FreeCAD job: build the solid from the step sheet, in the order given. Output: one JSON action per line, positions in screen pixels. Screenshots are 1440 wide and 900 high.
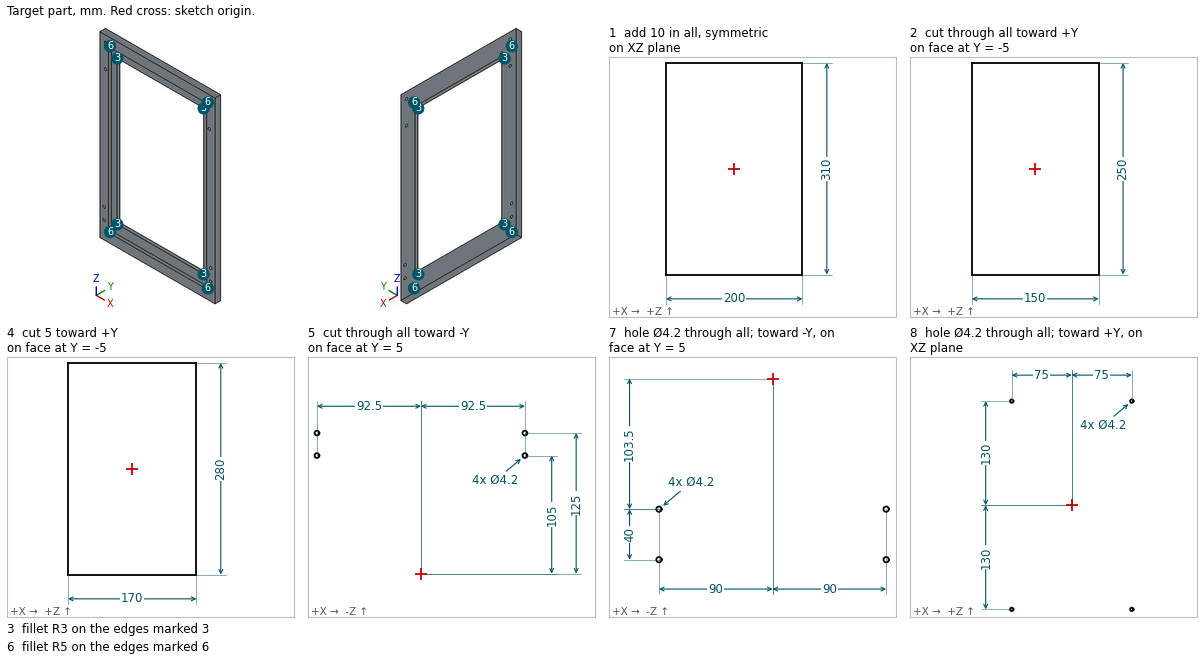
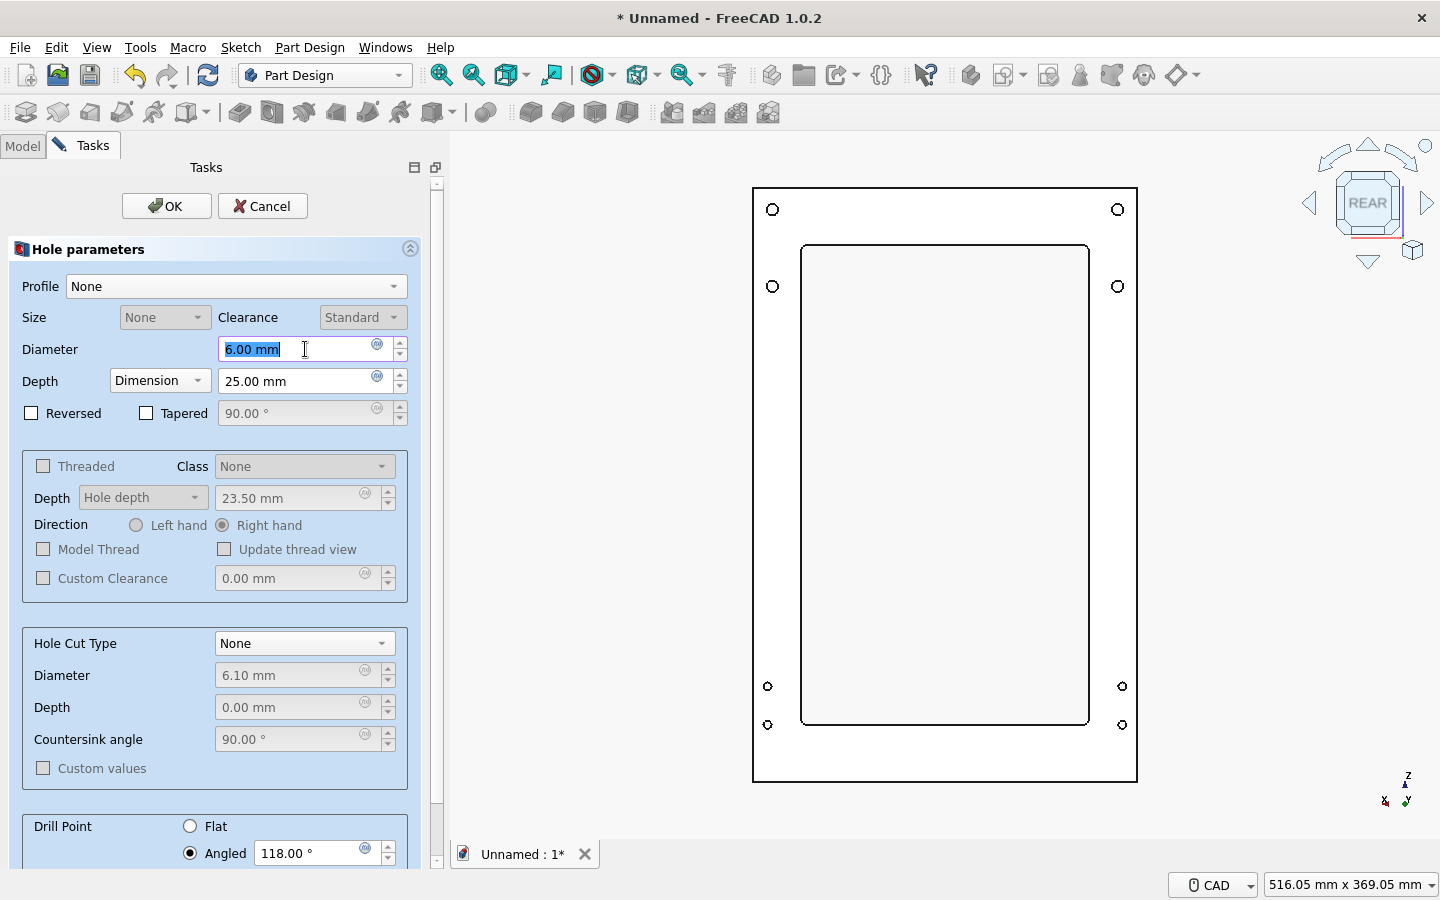
{"action": "type", "text": "4.2"}
{"action": "key", "text": "Tab"}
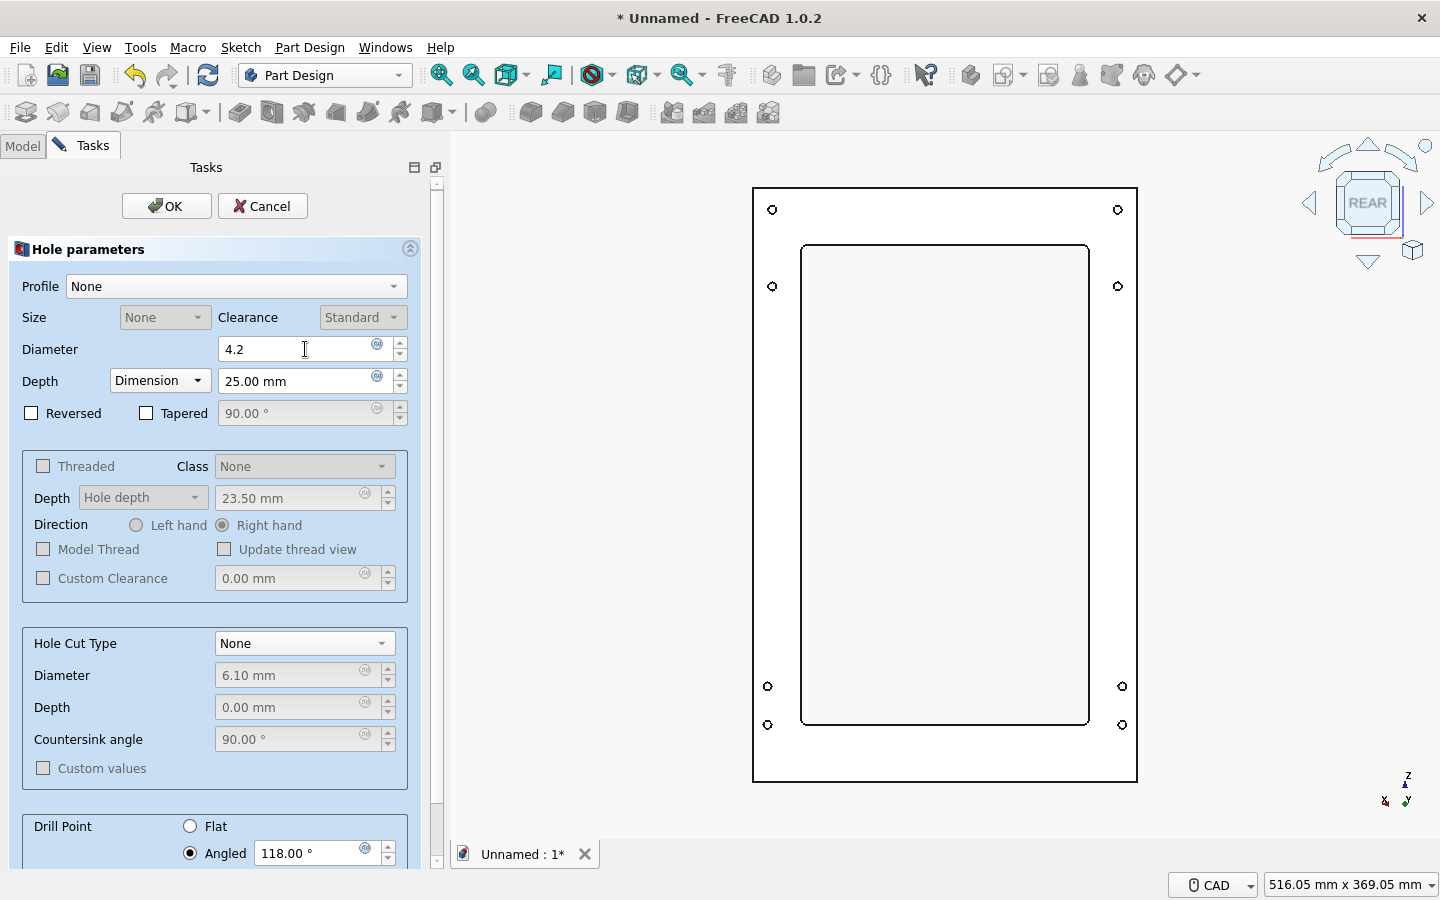
{"action": "left_click", "coordinate": [161, 380]}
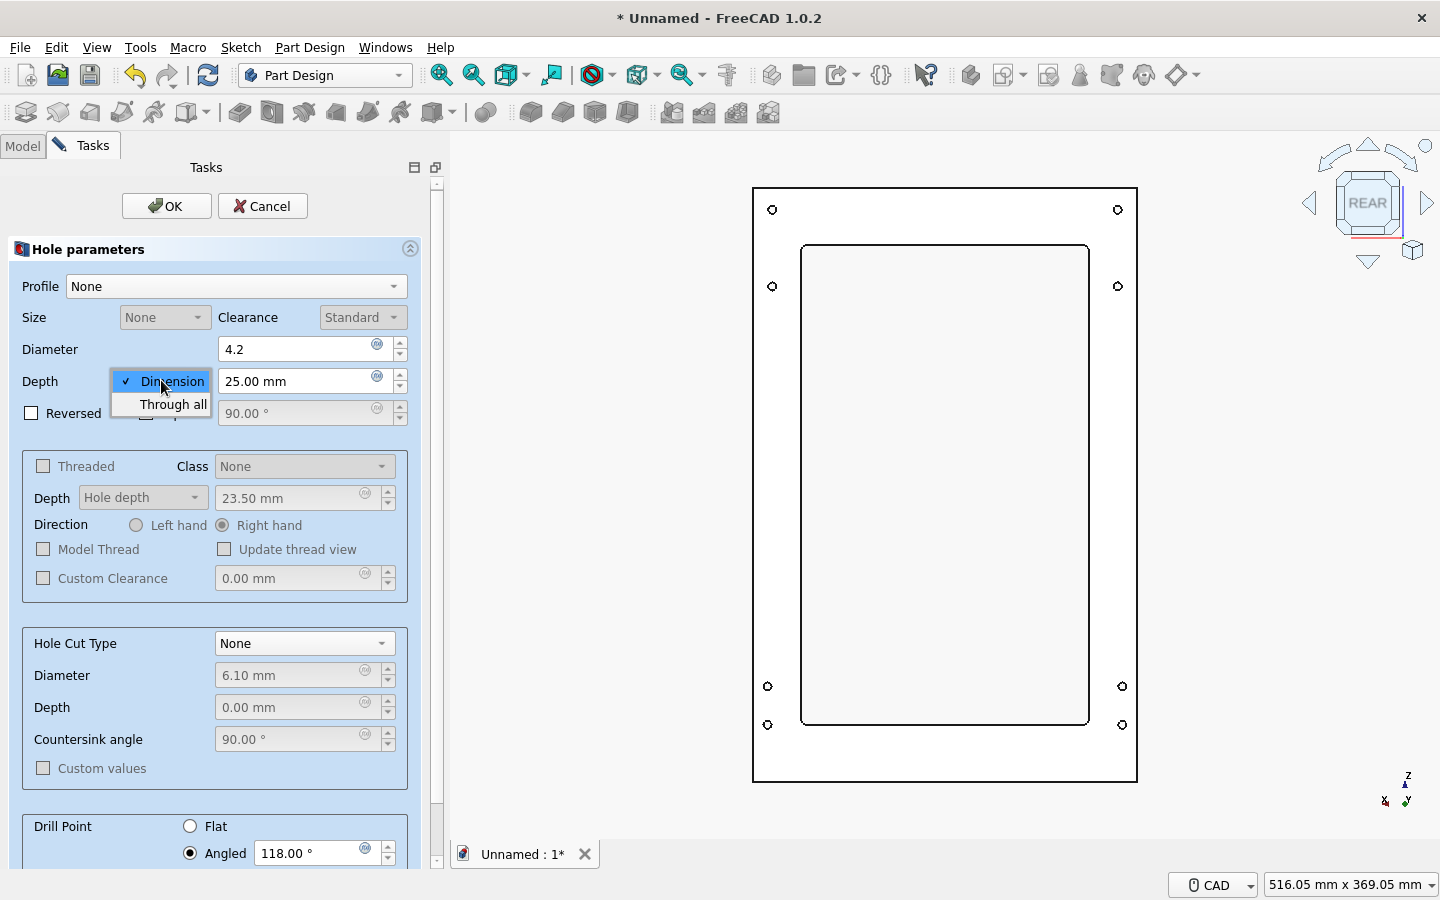
{"action": "left_click", "coordinate": [160, 404]}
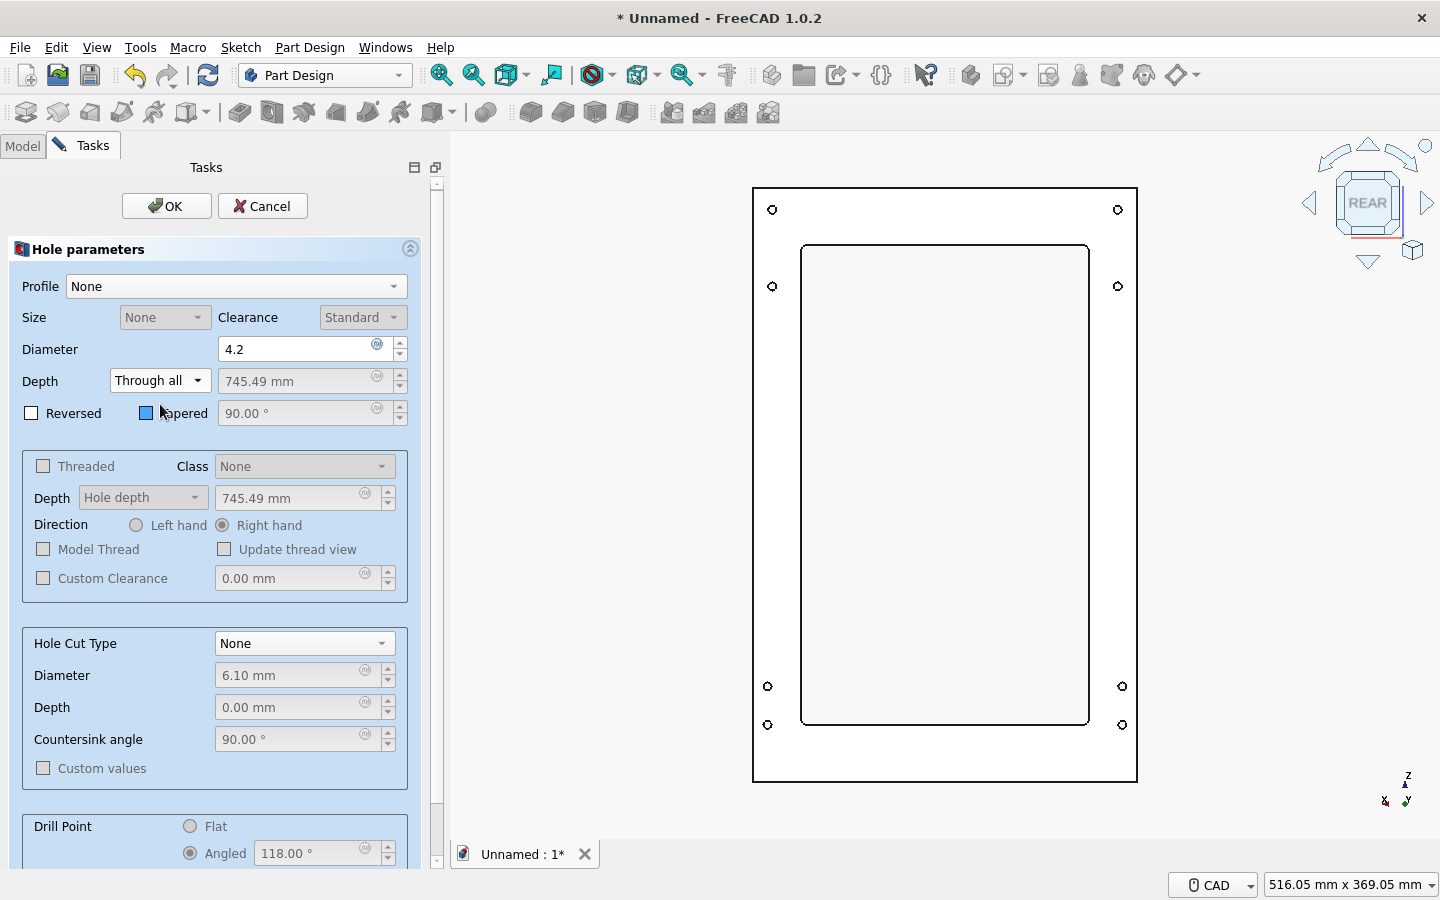
{"action": "left_click", "coordinate": [167, 206]}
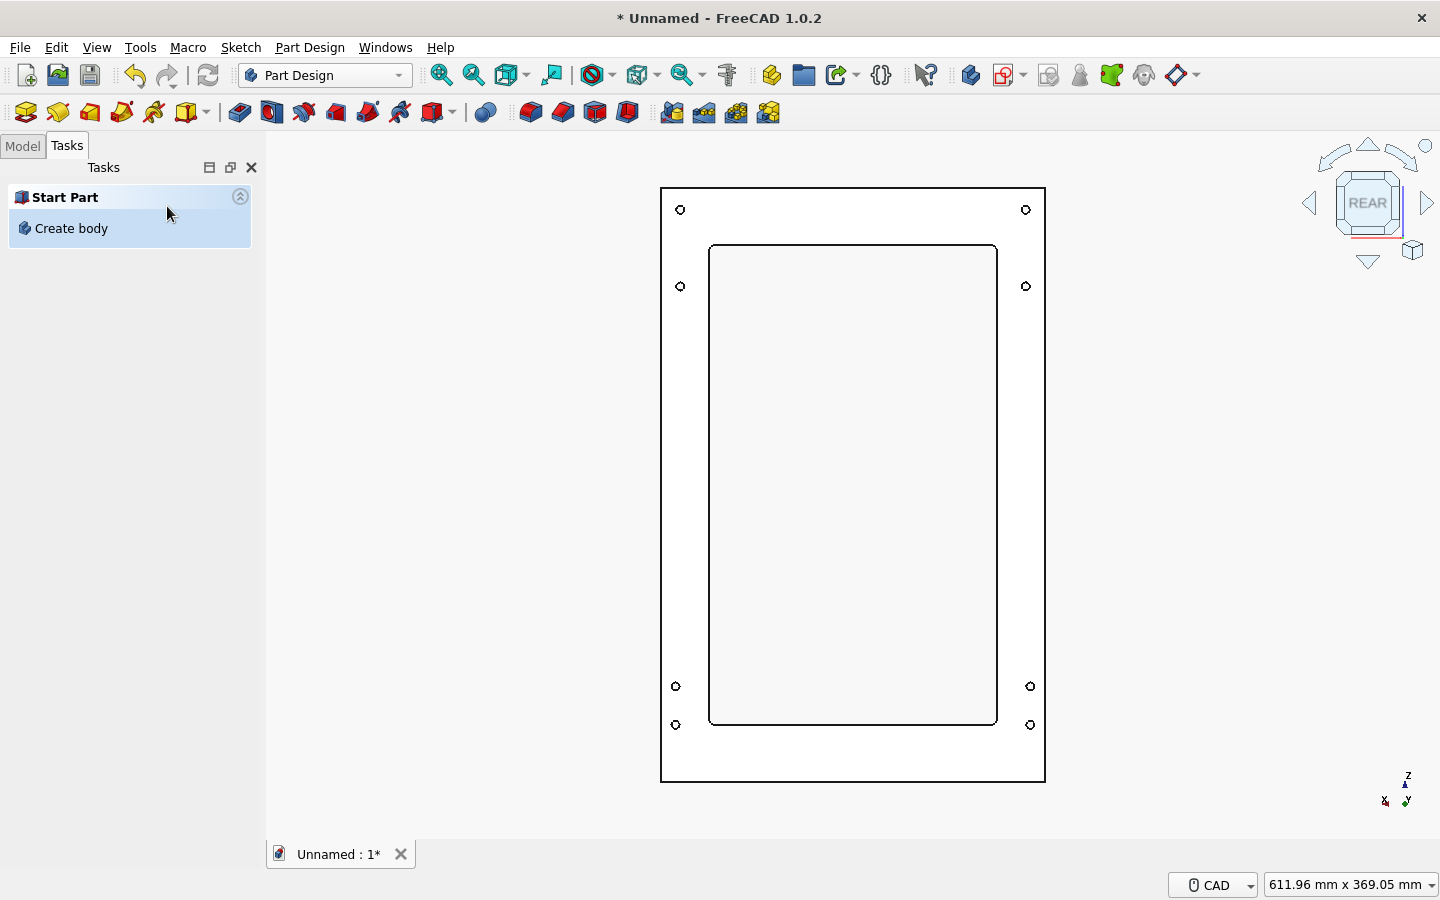
{"action": "left_click", "coordinate": [1004, 76]}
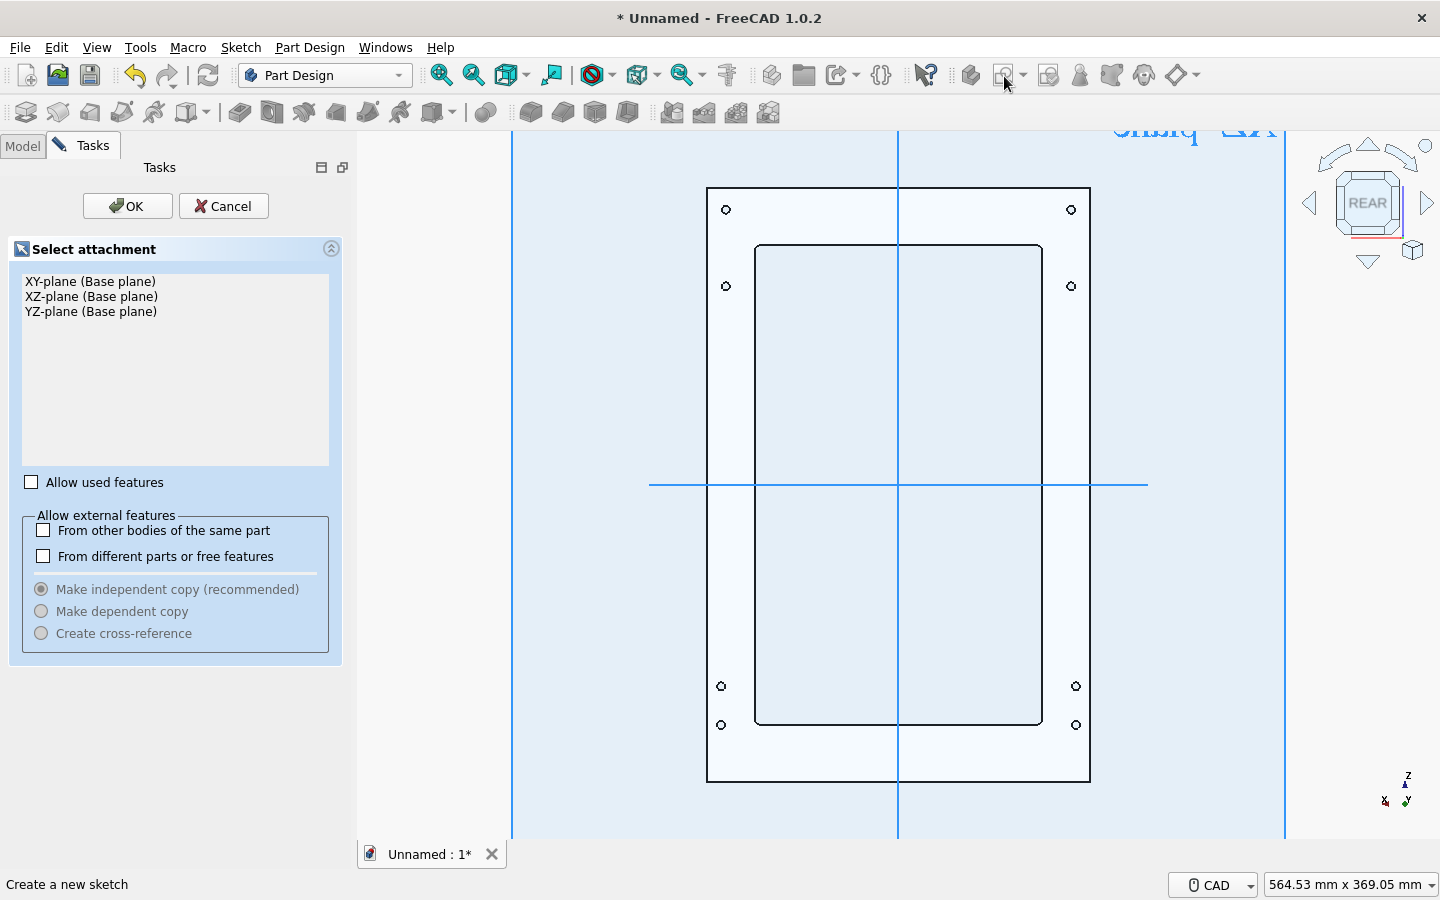
{"action": "left_click", "coordinate": [82, 296]}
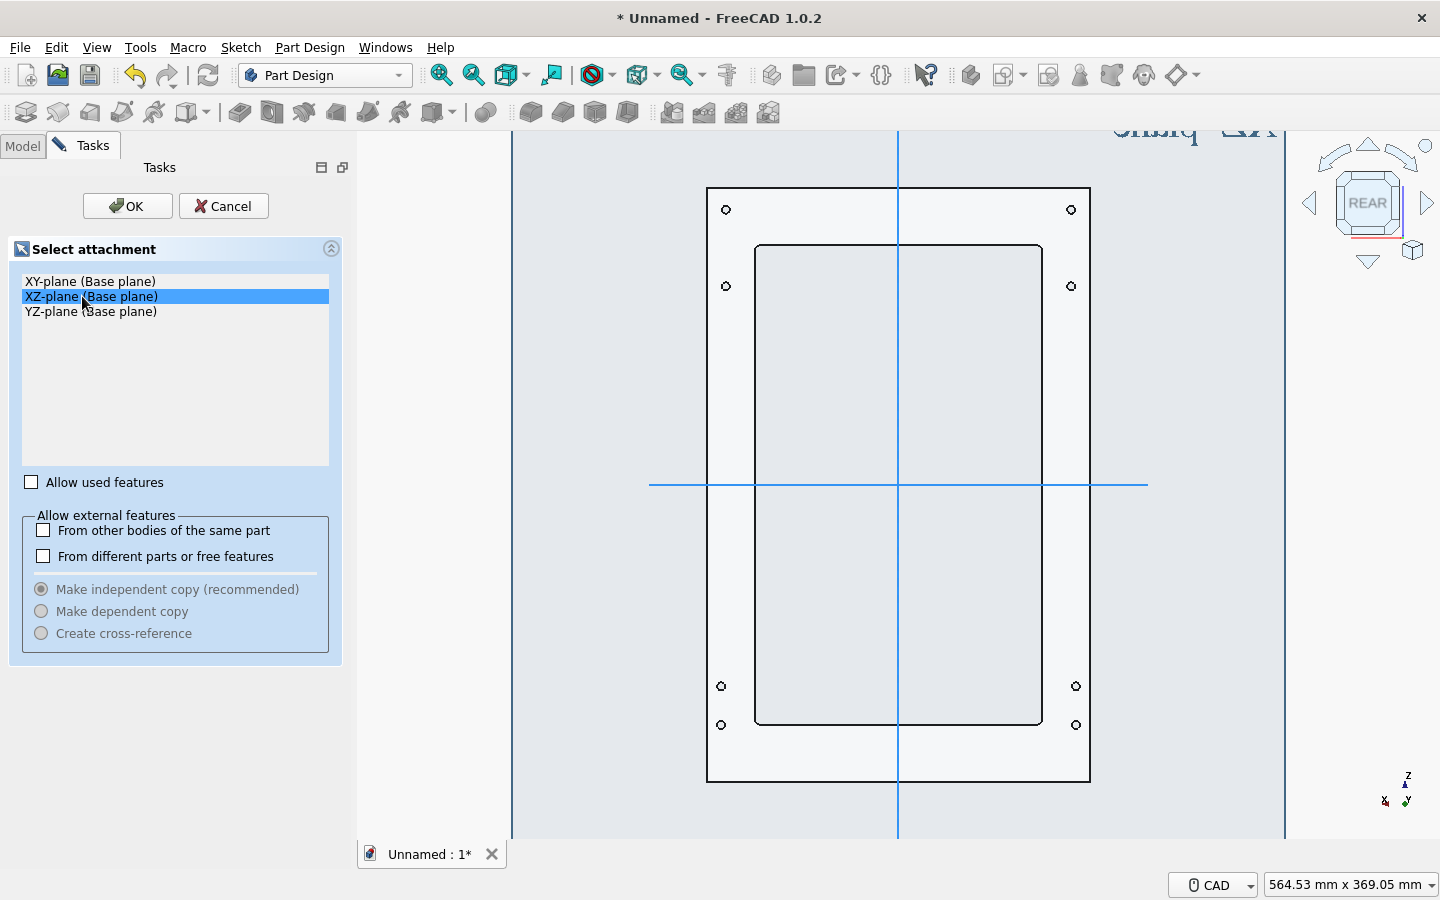
{"action": "left_click", "coordinate": [128, 206]}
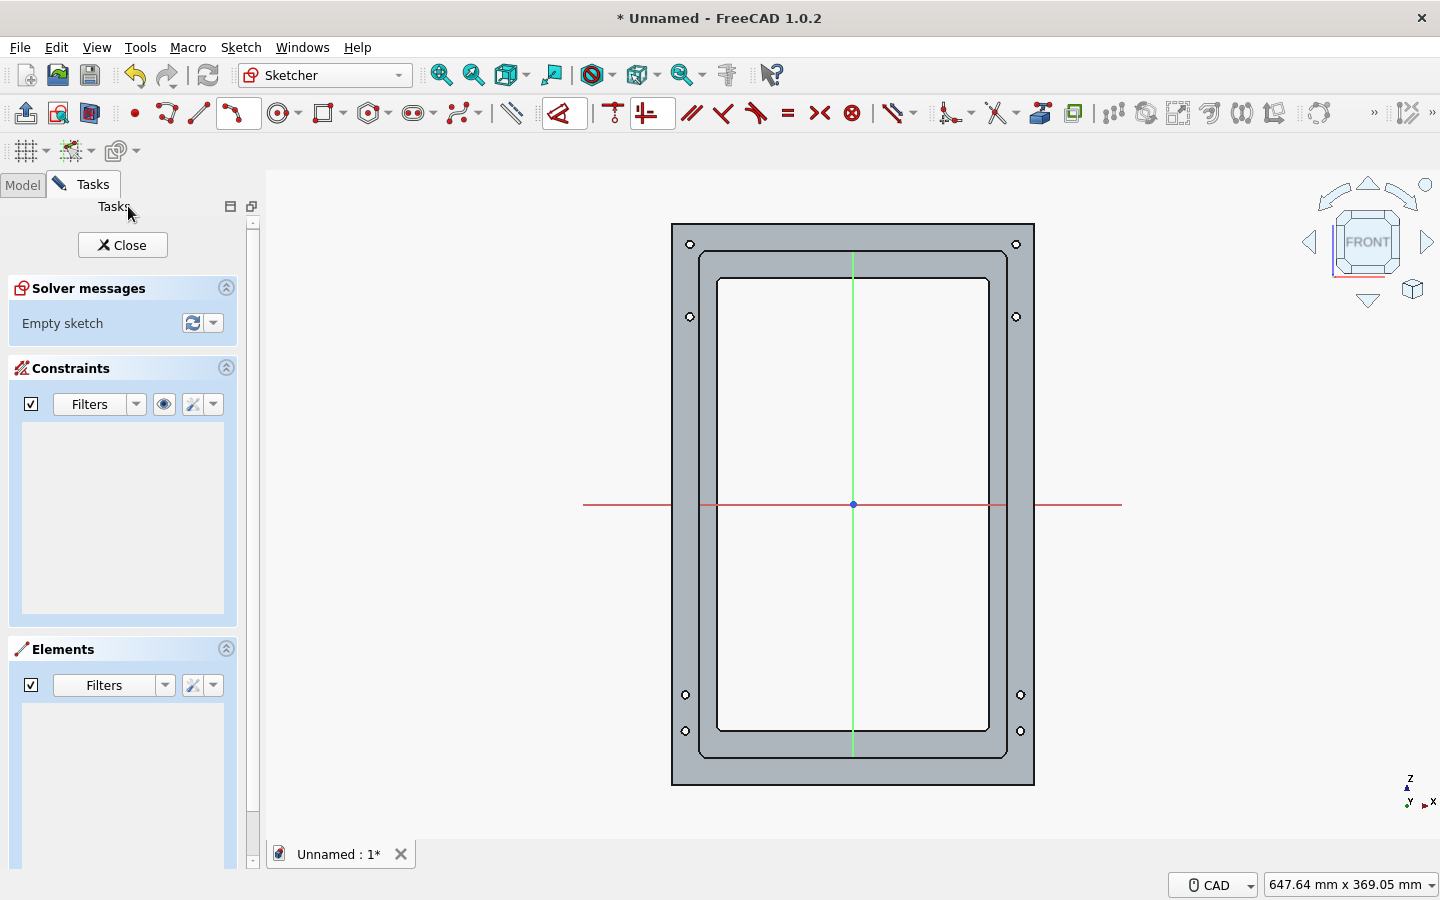
{"action": "key", "text": "q s"}